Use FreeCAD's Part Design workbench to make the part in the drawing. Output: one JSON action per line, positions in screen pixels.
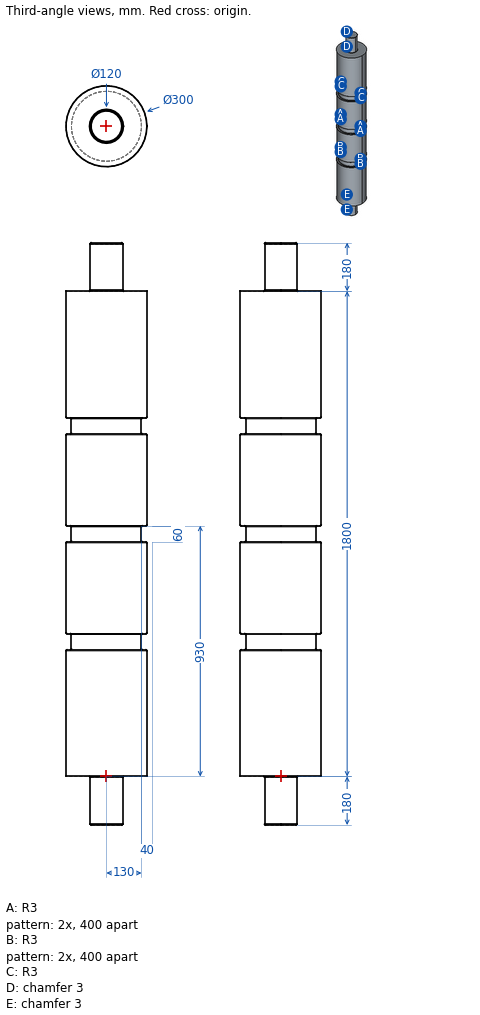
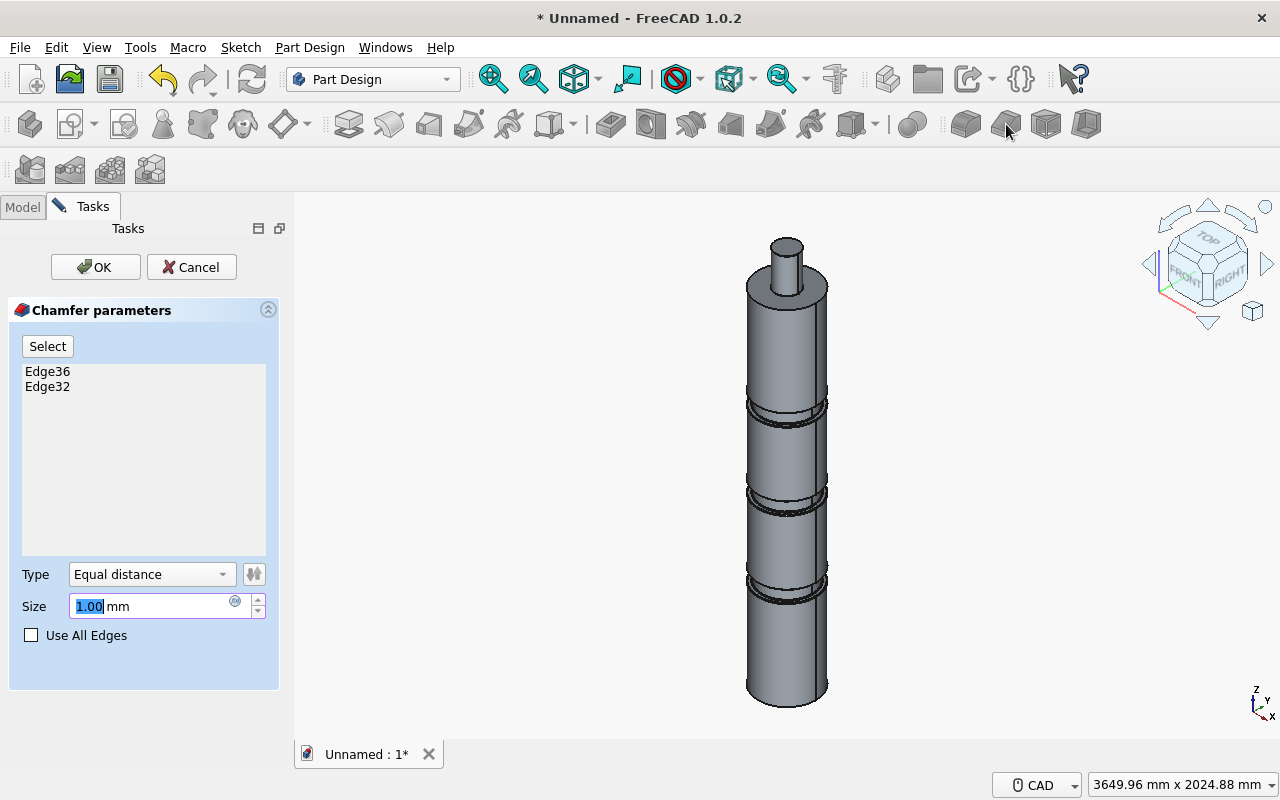
{"action": "type", "text": "3"}
{"action": "key", "text": "Tab"}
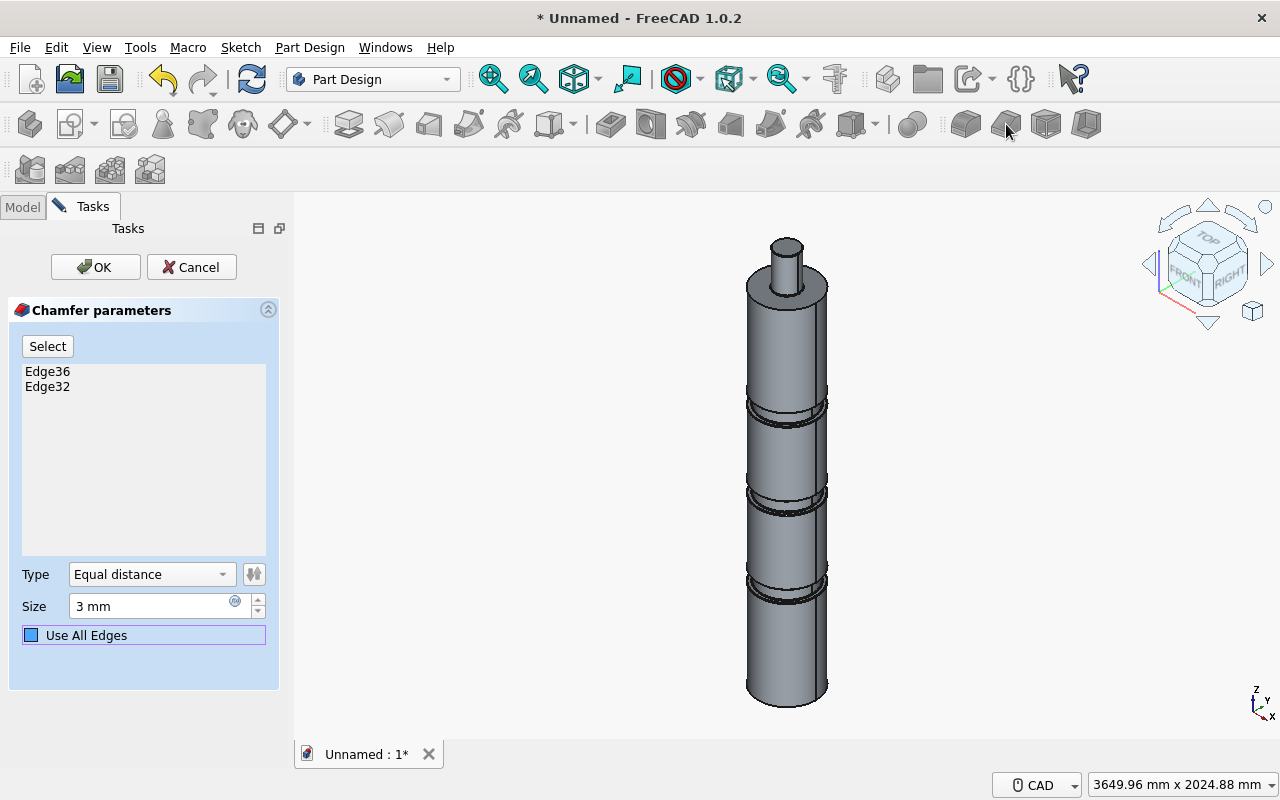
{"action": "left_click", "coordinate": [96, 267]}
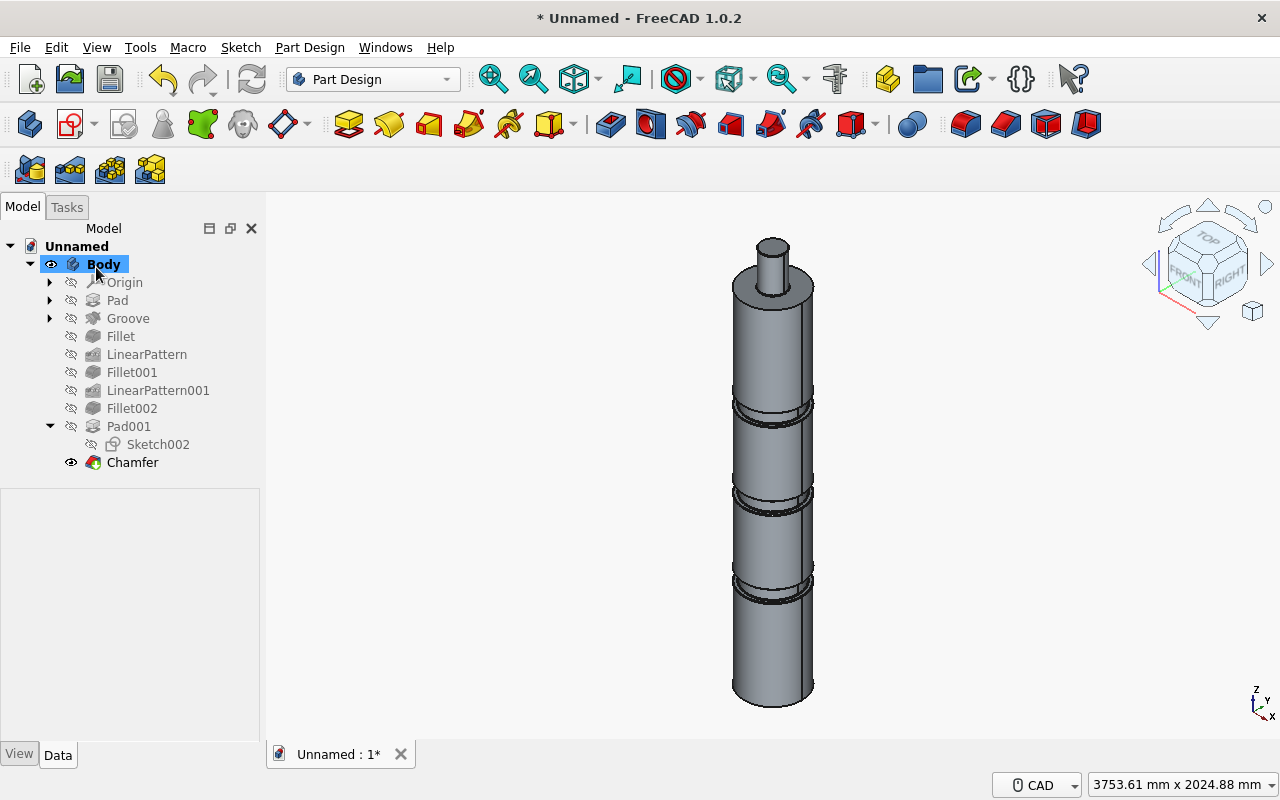
{"action": "left_click", "coordinate": [50, 282]}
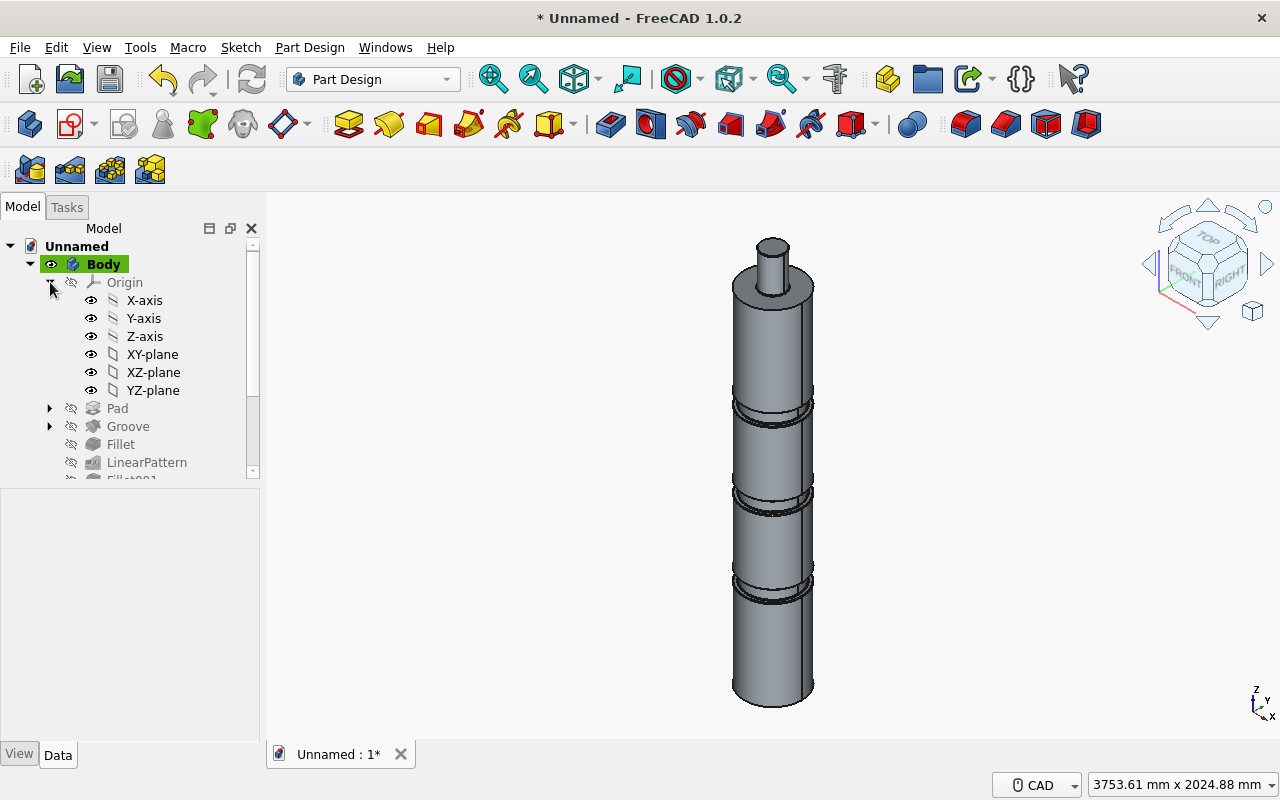
{"action": "left_click", "coordinate": [136, 354]}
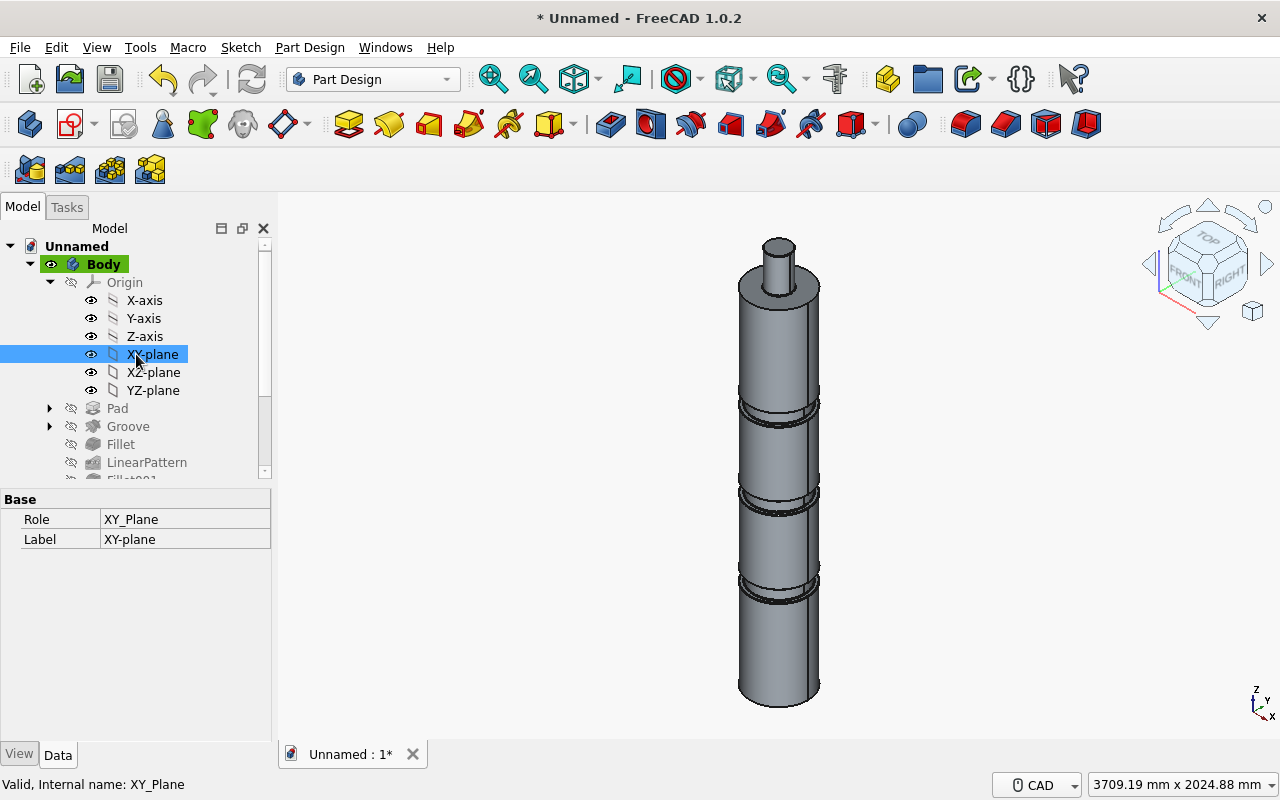
{"action": "left_click", "coordinate": [284, 124]}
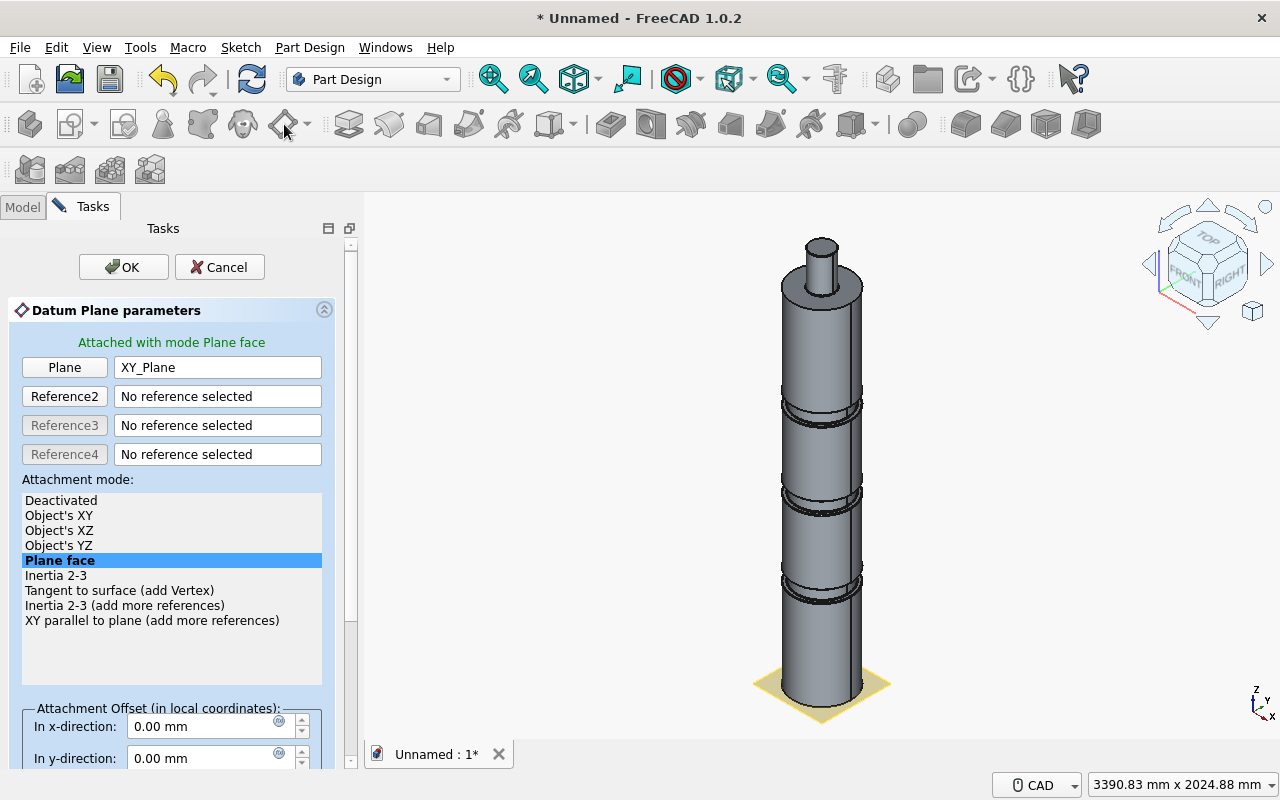
{"action": "scroll", "coordinate": [351, 503], "scroll_direction": "down", "scroll_amount": 2}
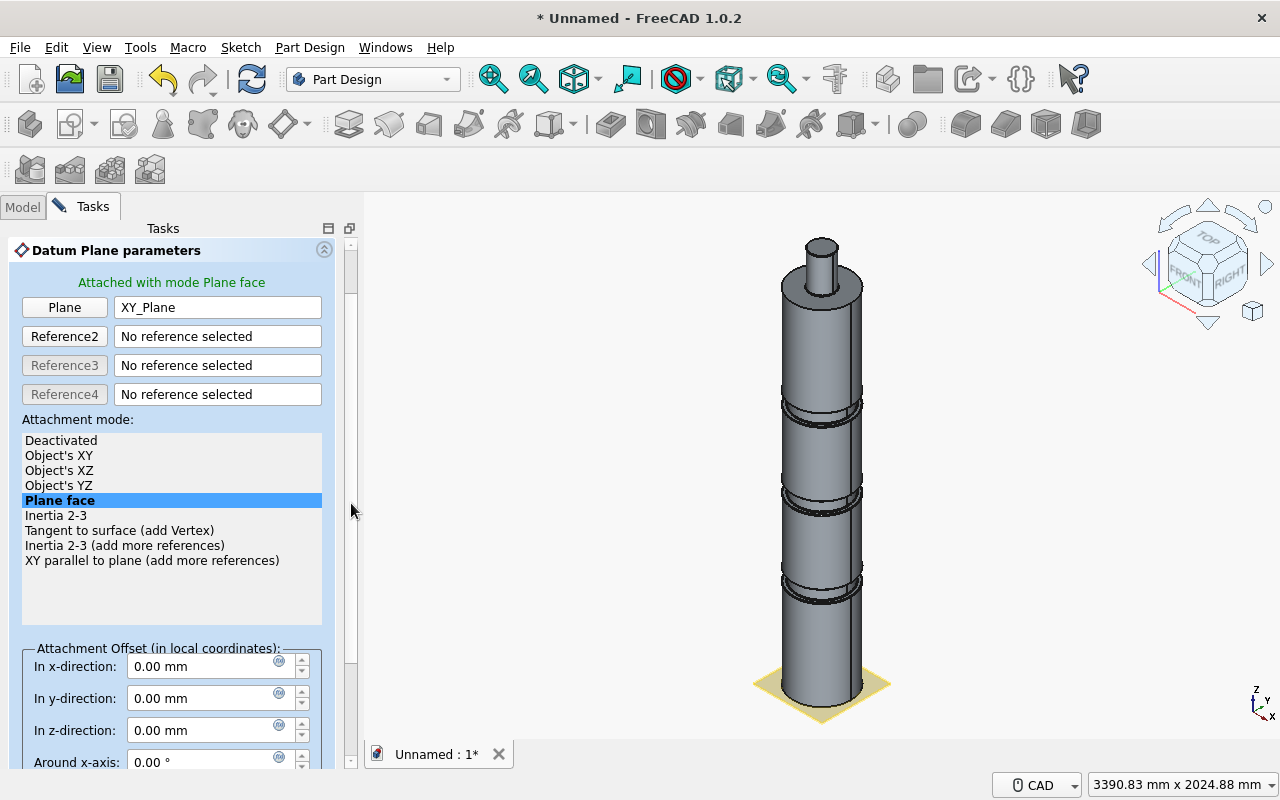
{"action": "triple_click", "coordinate": [210, 670]}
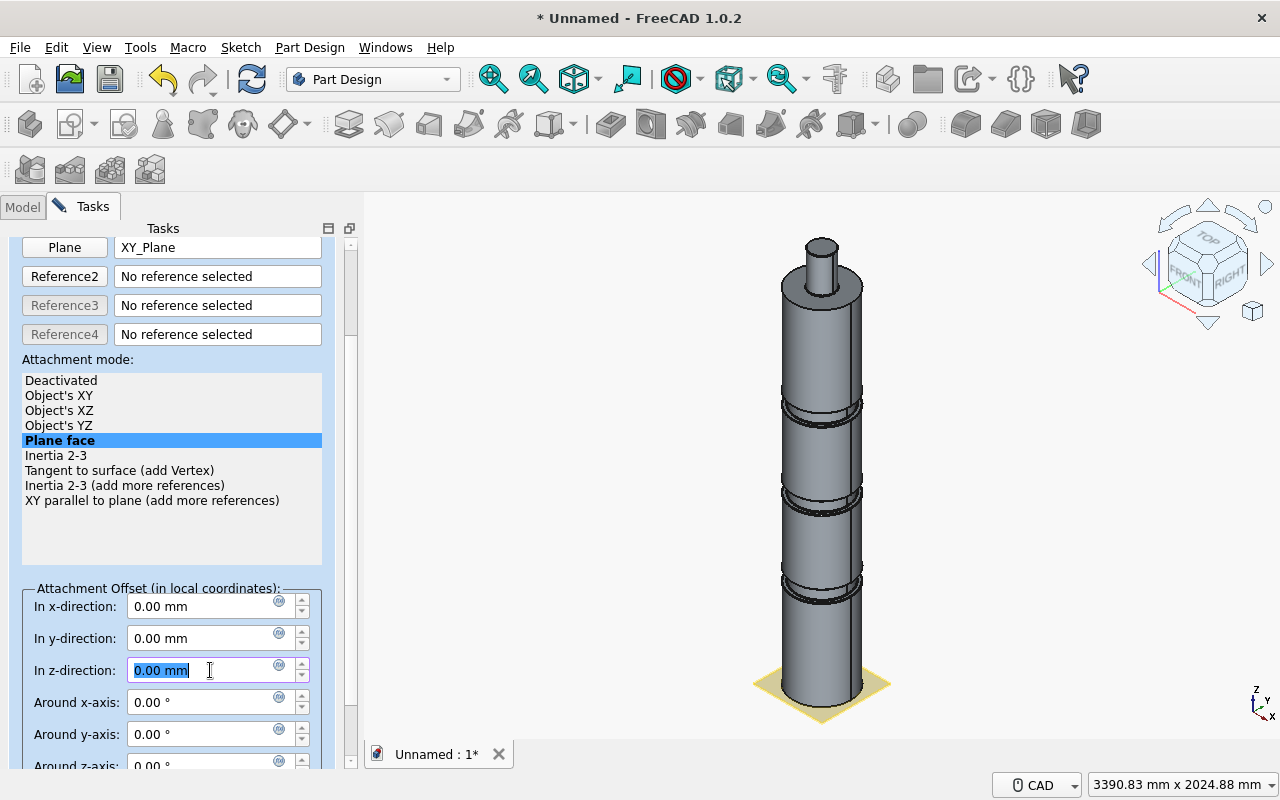
{"action": "type", "text": "-180"}
{"action": "key", "text": "Tab"}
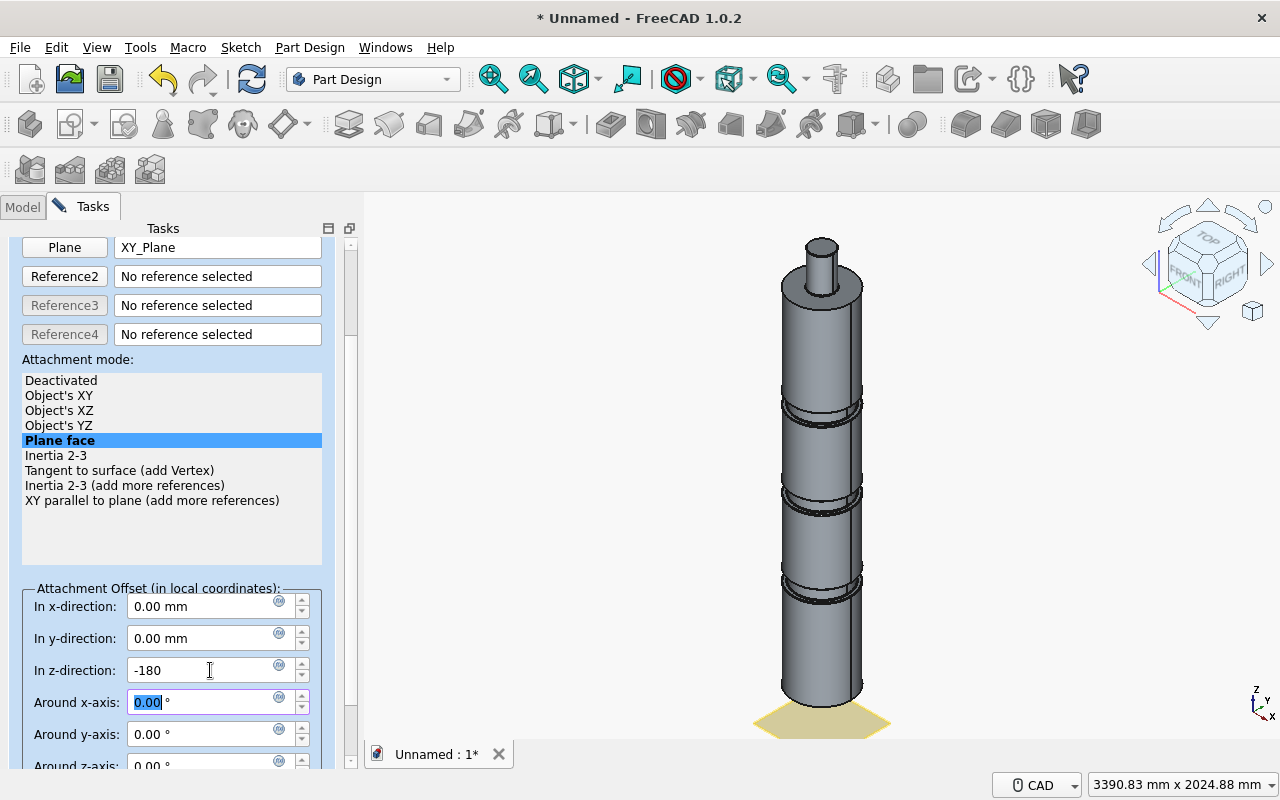
{"action": "scroll", "coordinate": [351, 503], "scroll_direction": "up", "scroll_amount": 3}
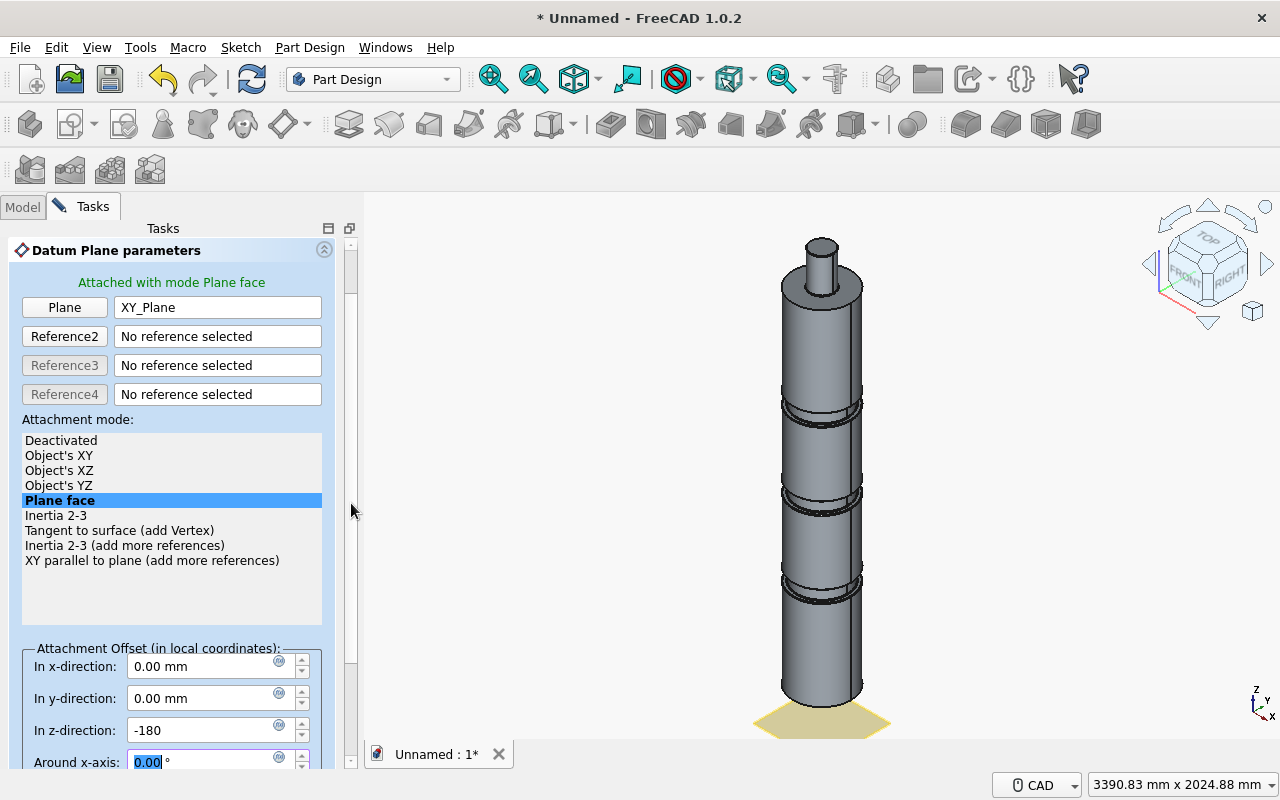
{"action": "left_click", "coordinate": [124, 267]}